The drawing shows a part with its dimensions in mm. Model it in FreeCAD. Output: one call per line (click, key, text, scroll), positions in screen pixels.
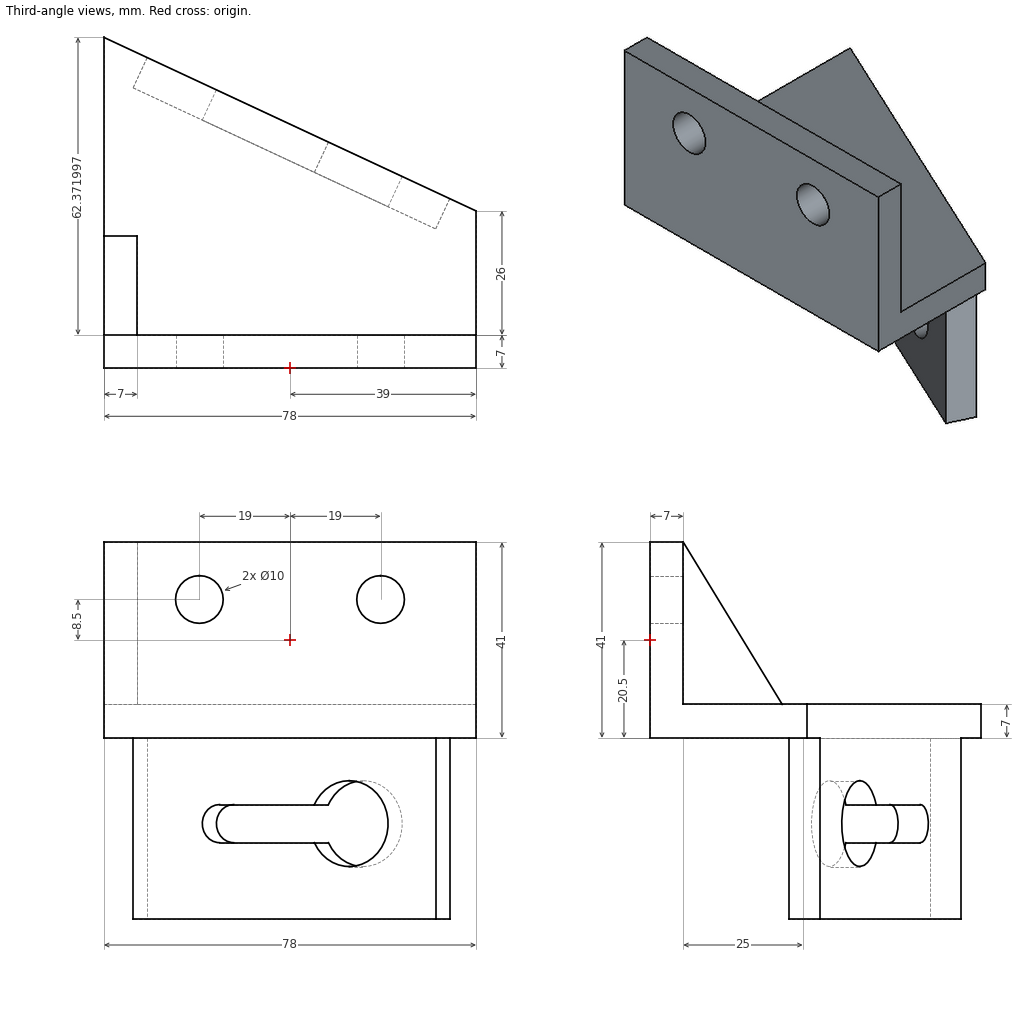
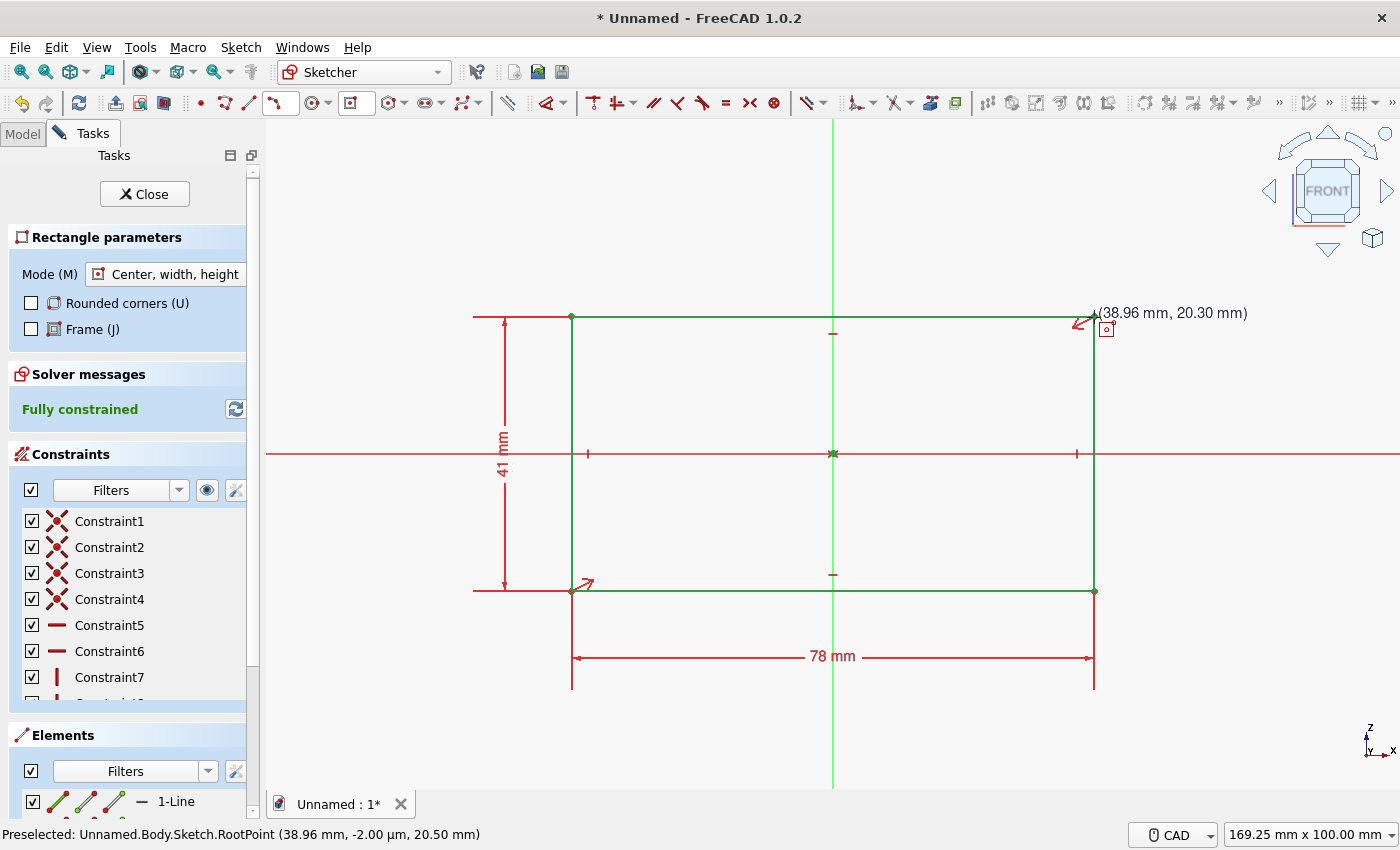
click(312, 104)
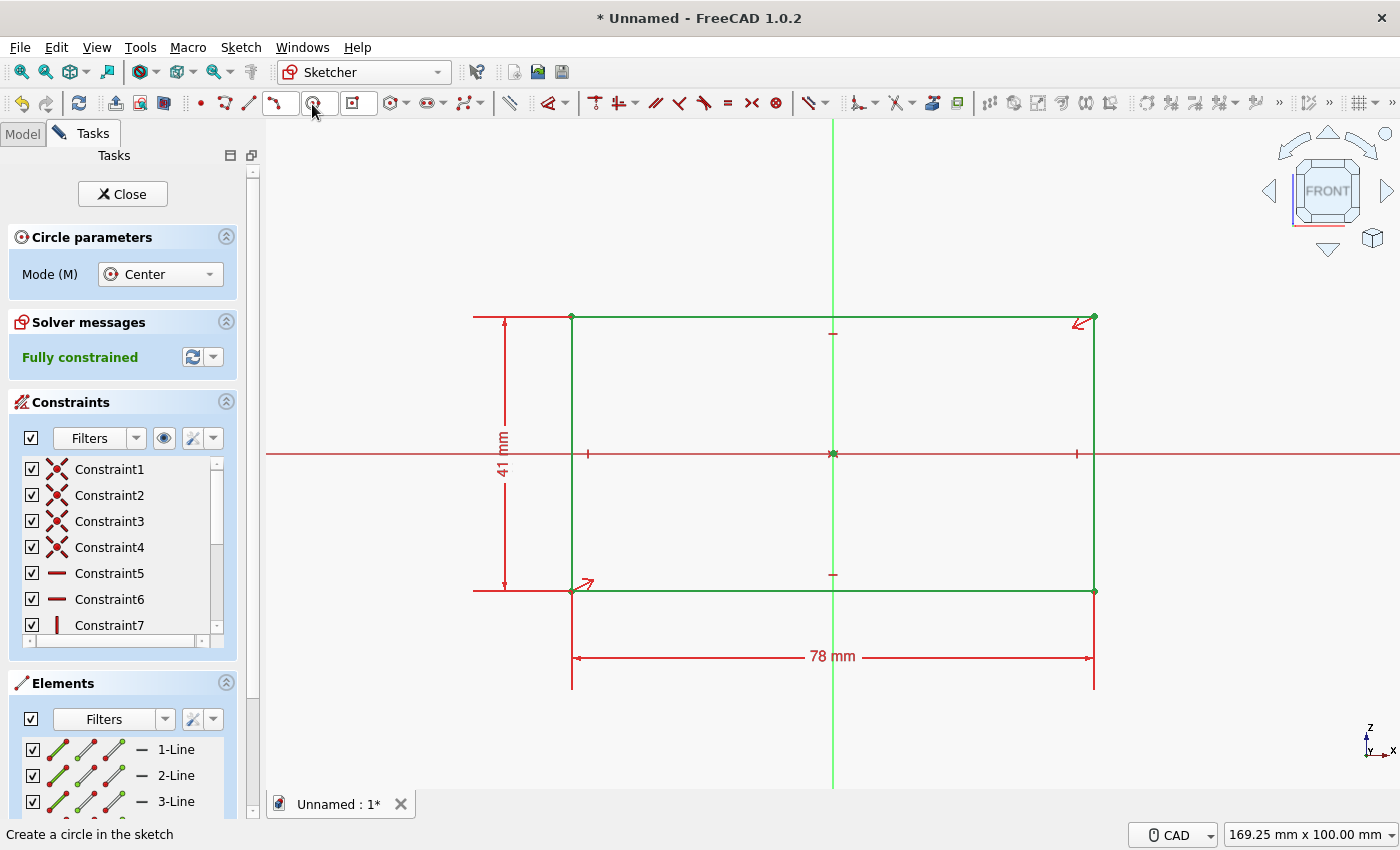
click(706, 397)
move(729, 373)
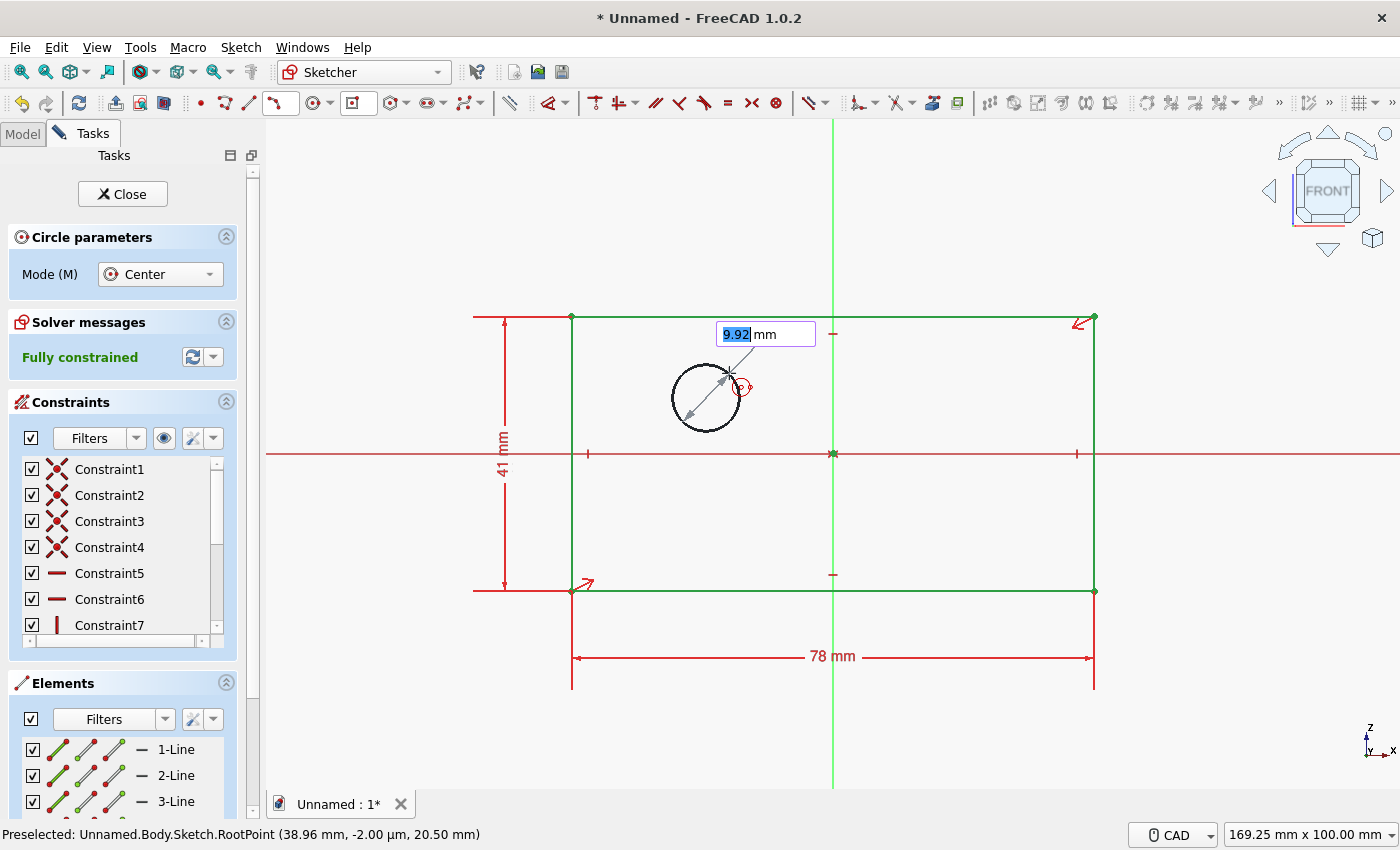
text(10)
key(Return)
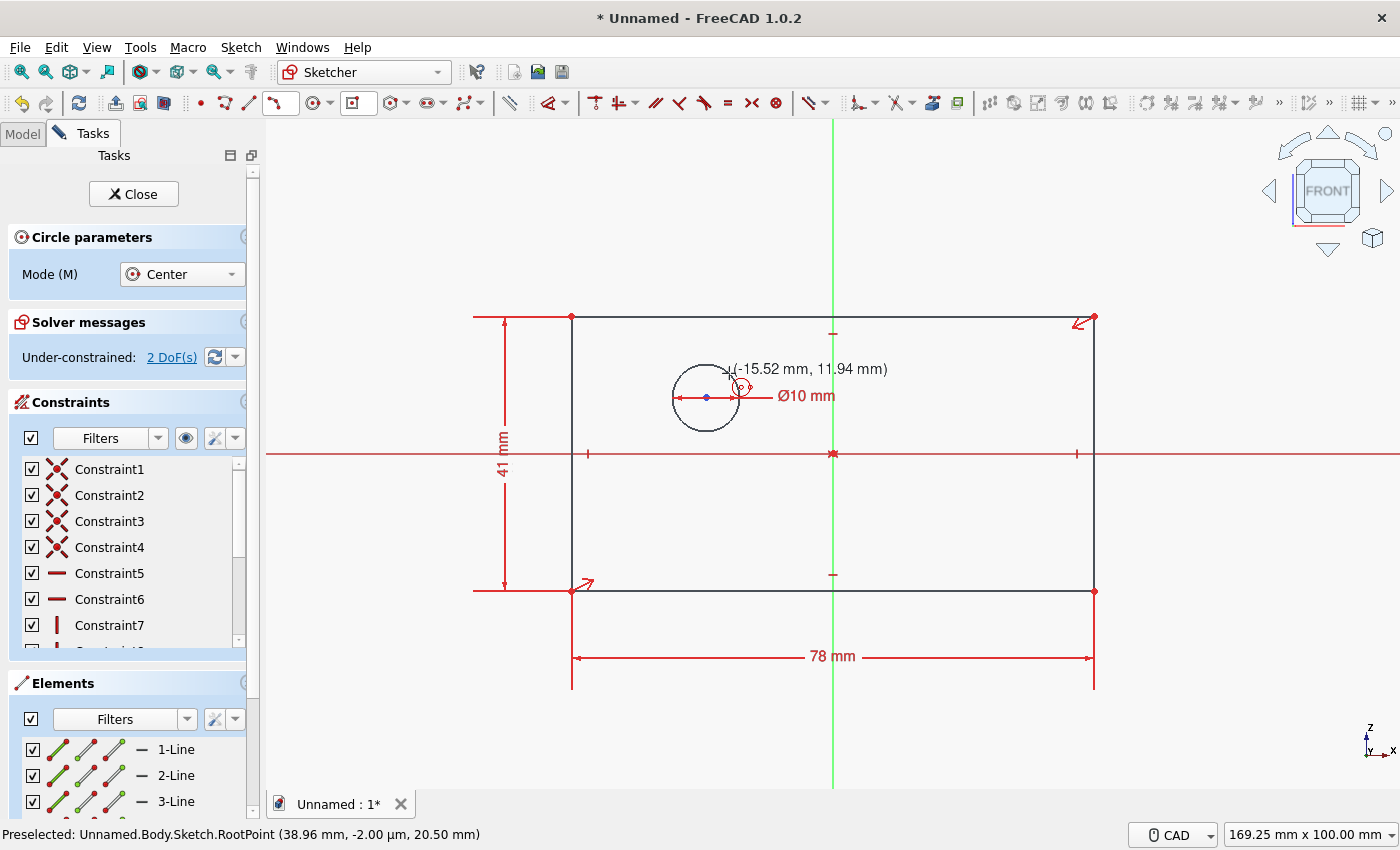
click(960, 397)
move(984, 373)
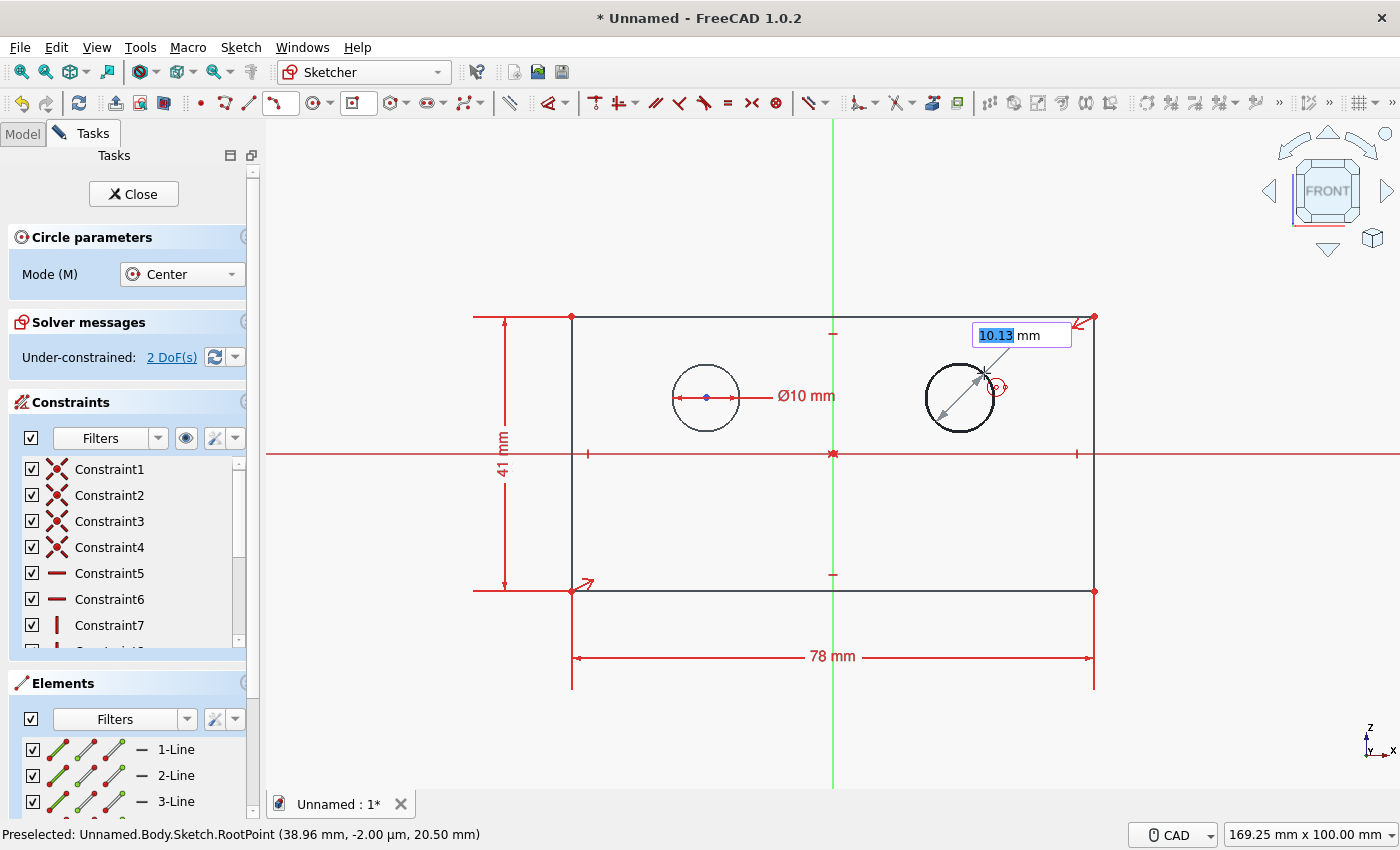
text(10)
key(Return)
key(Escape)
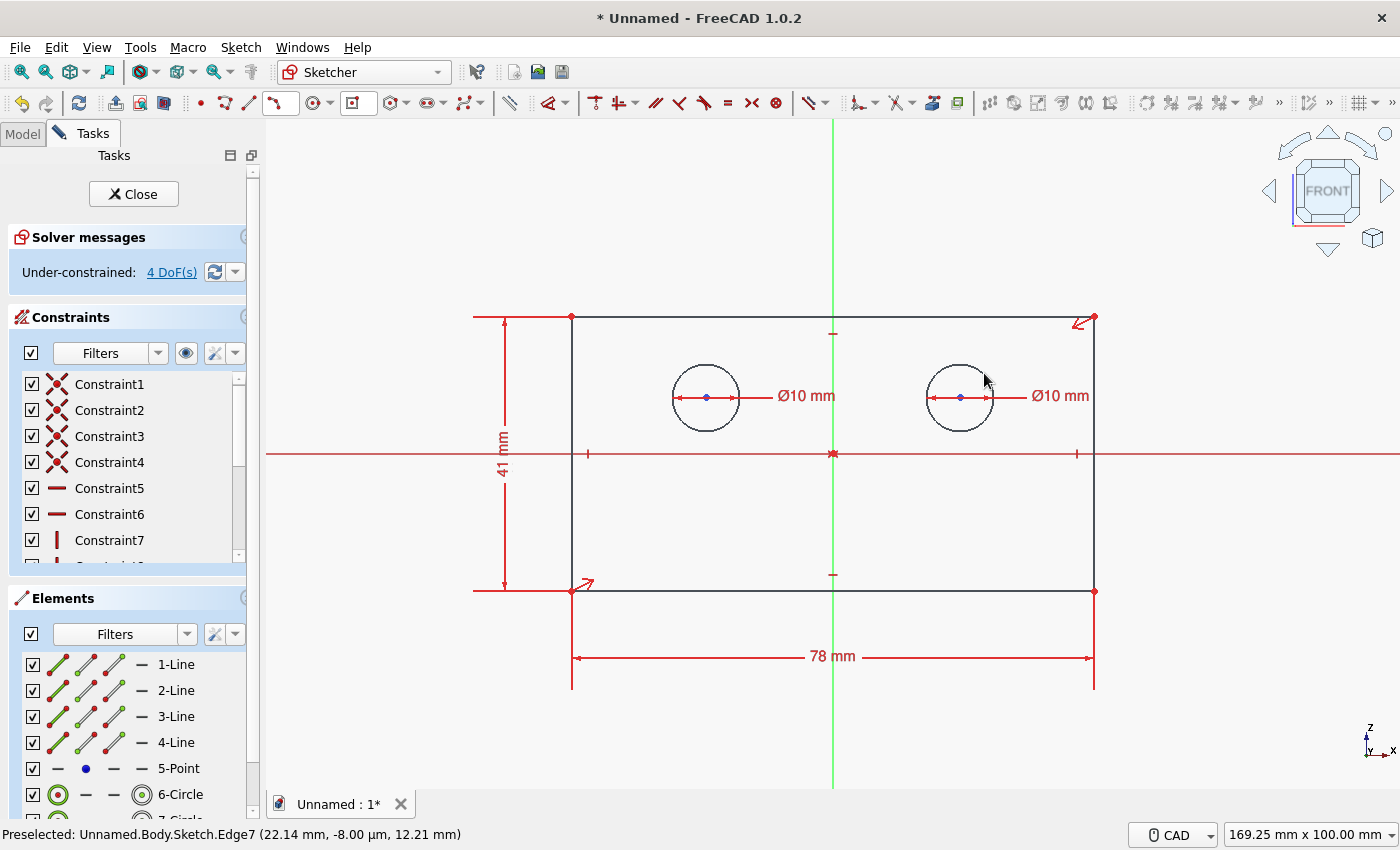
click(706, 398)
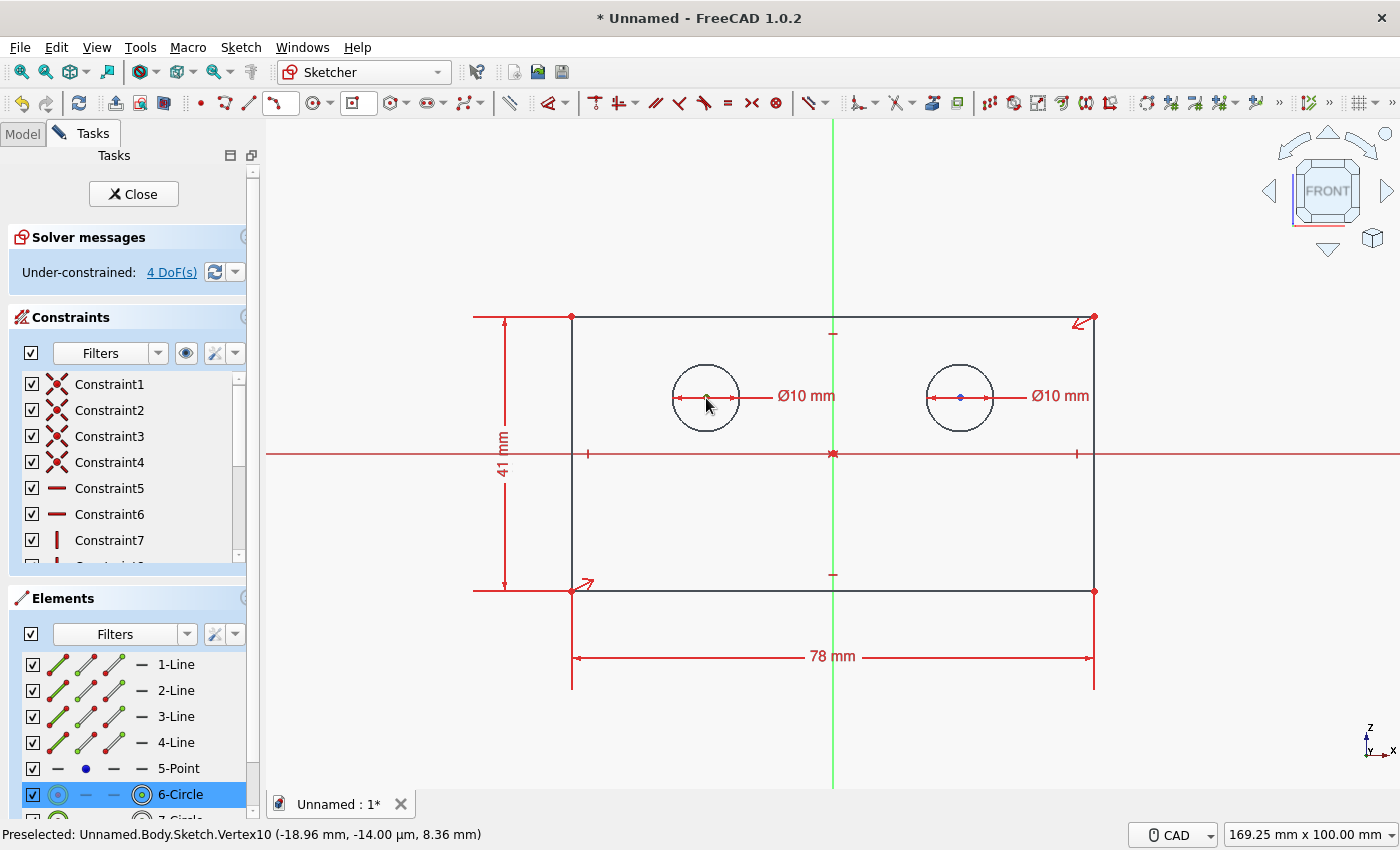
click(960, 398)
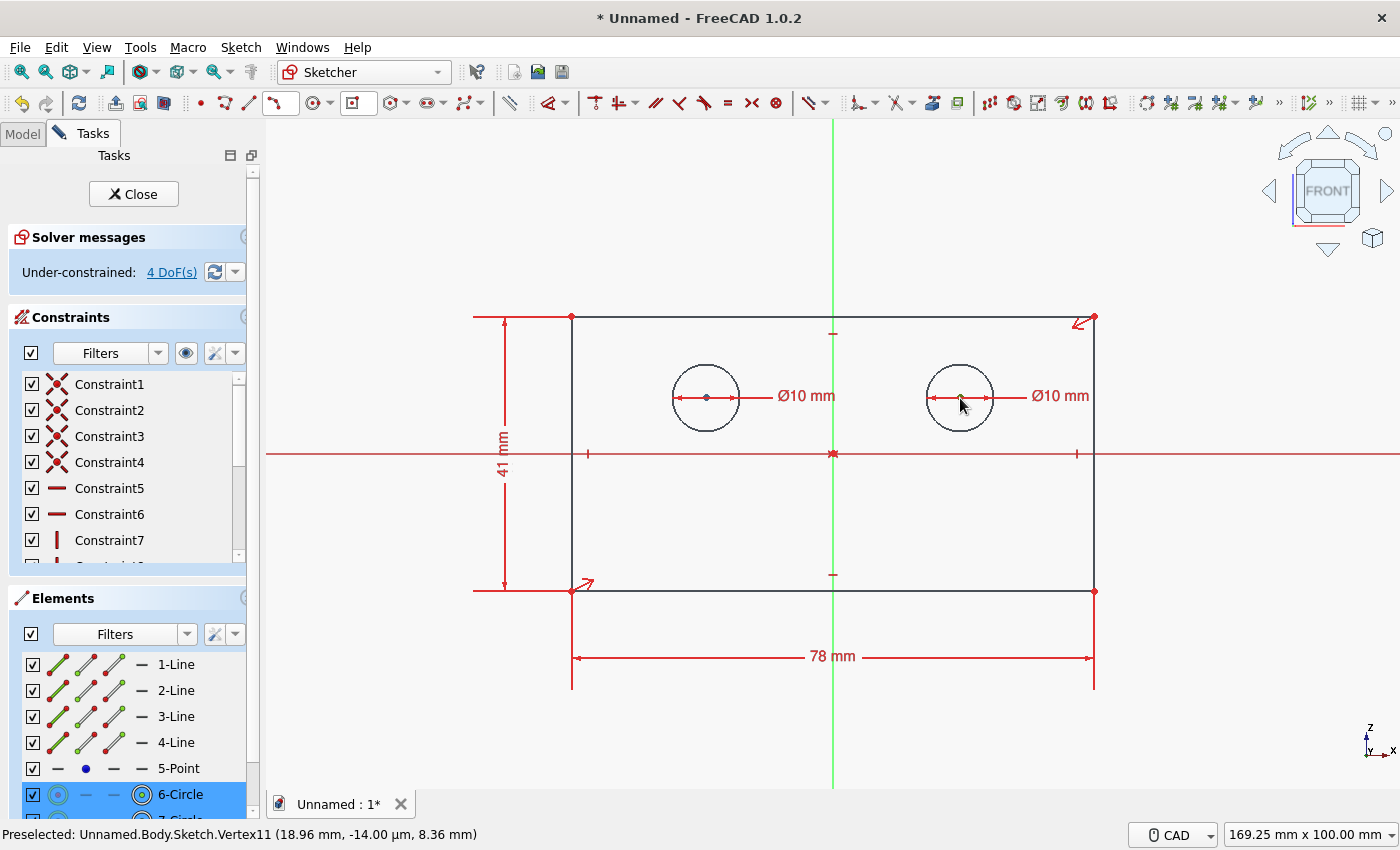
click(638, 104)